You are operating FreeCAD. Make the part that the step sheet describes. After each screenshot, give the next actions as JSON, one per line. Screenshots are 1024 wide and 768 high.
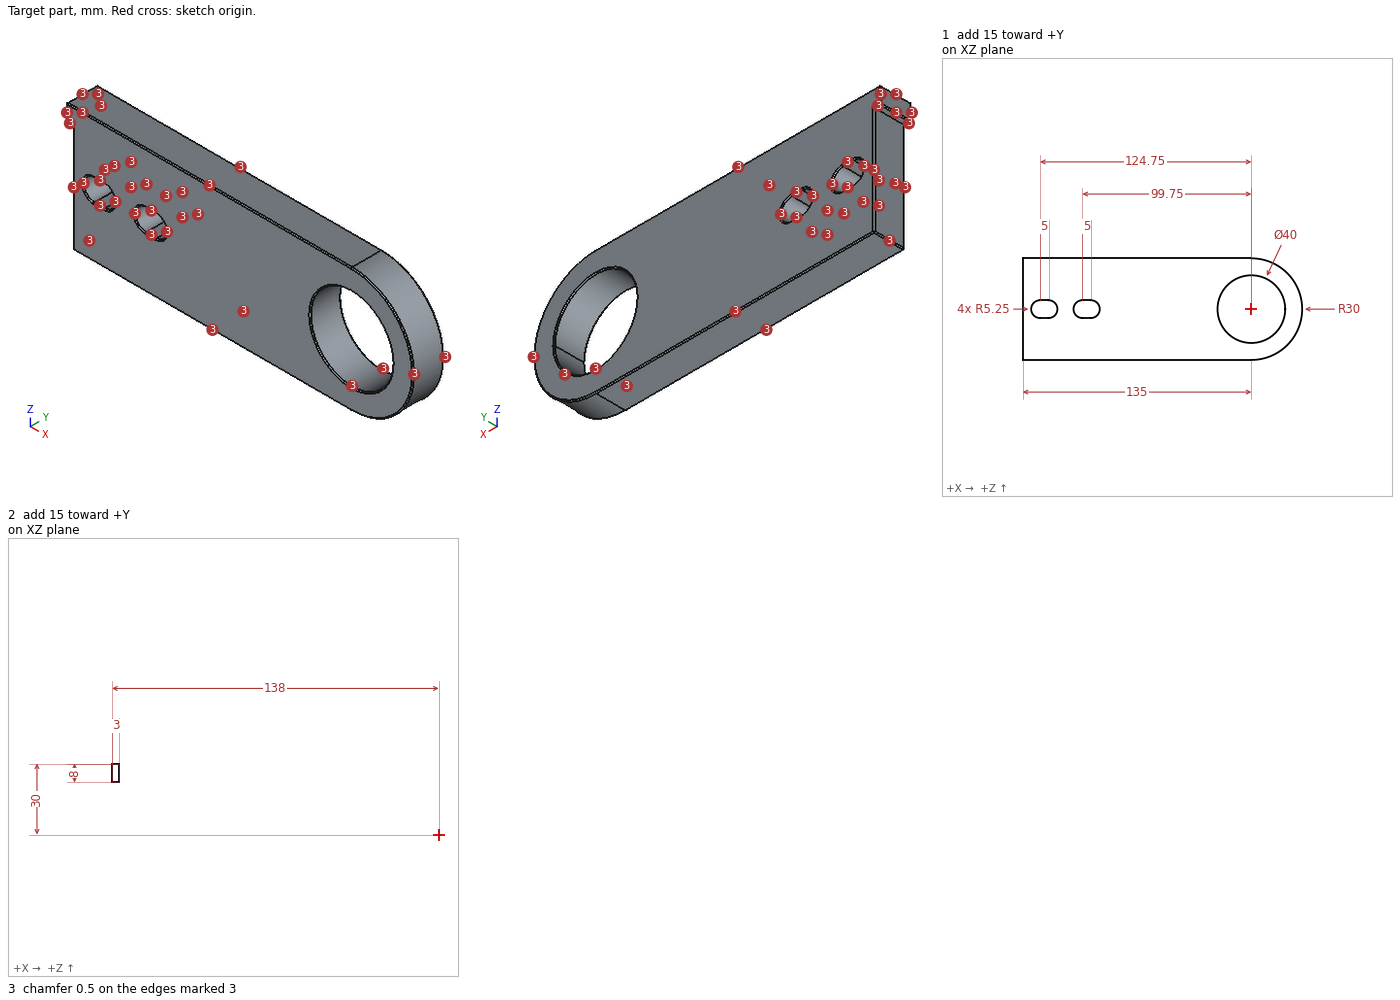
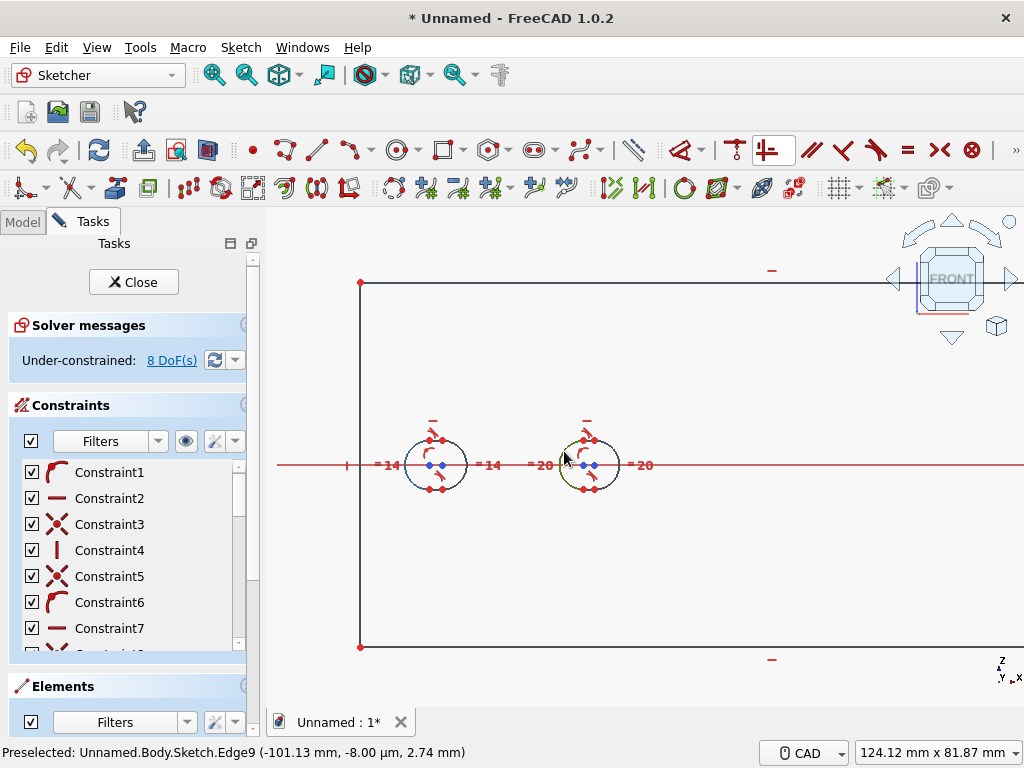
{"action": "left_click", "coordinate": [908, 150]}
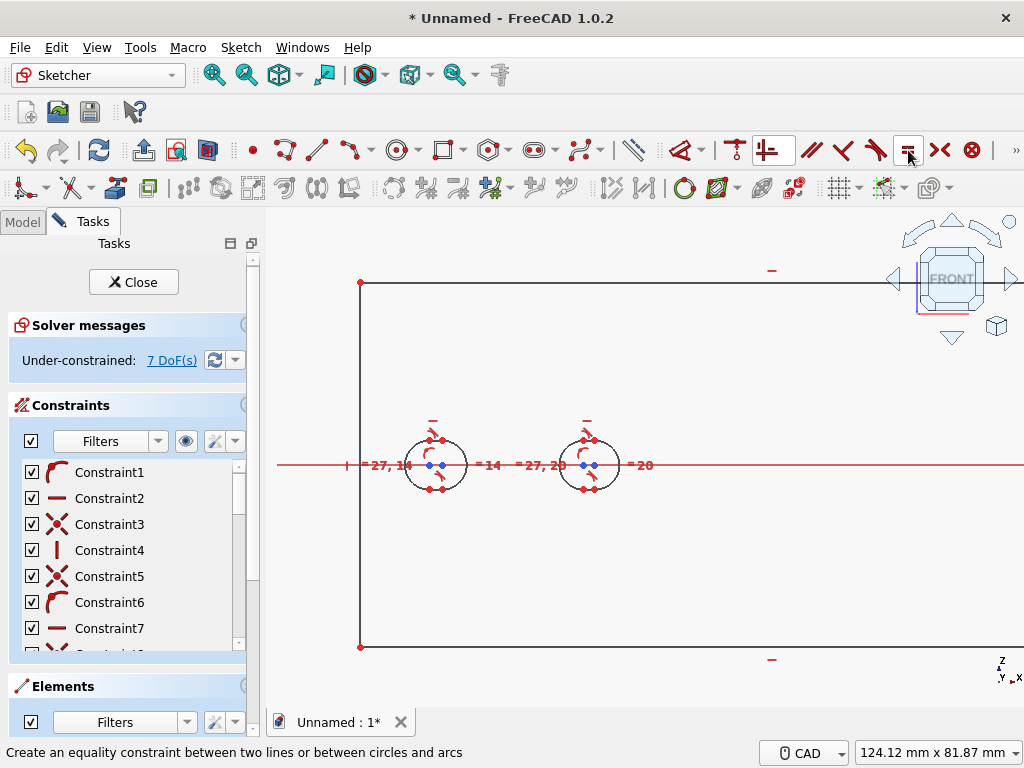
{"action": "left_click", "coordinate": [680, 150]}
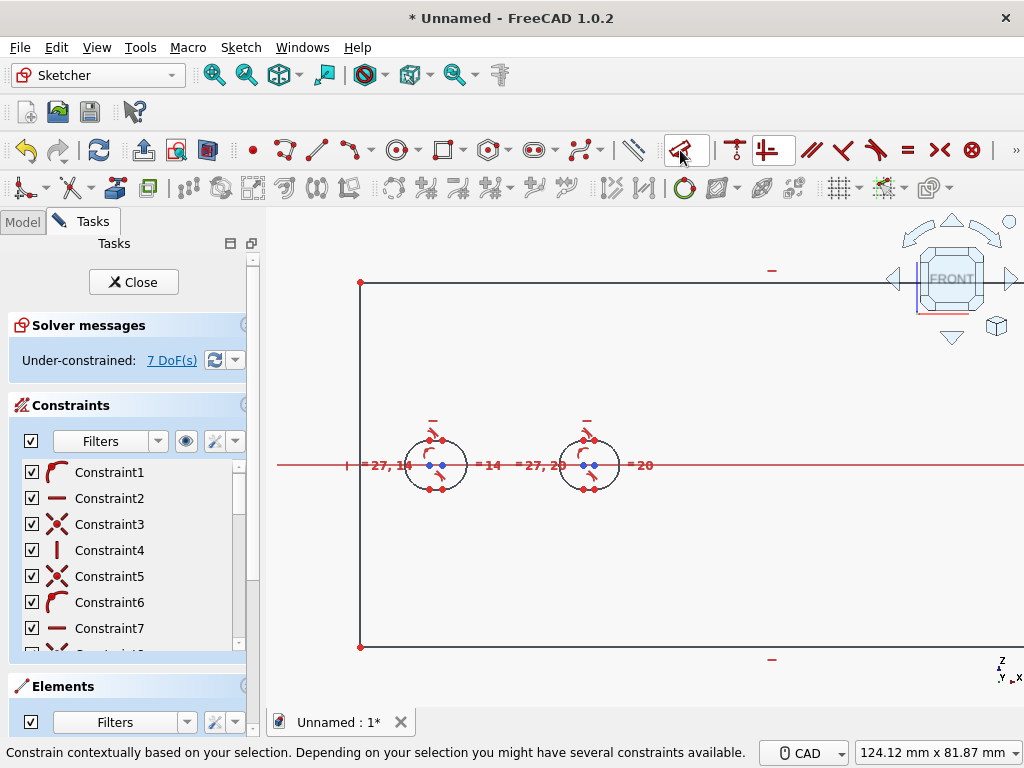
{"action": "scroll", "coordinate": [410, 452], "scroll_direction": "down", "scroll_amount": 5}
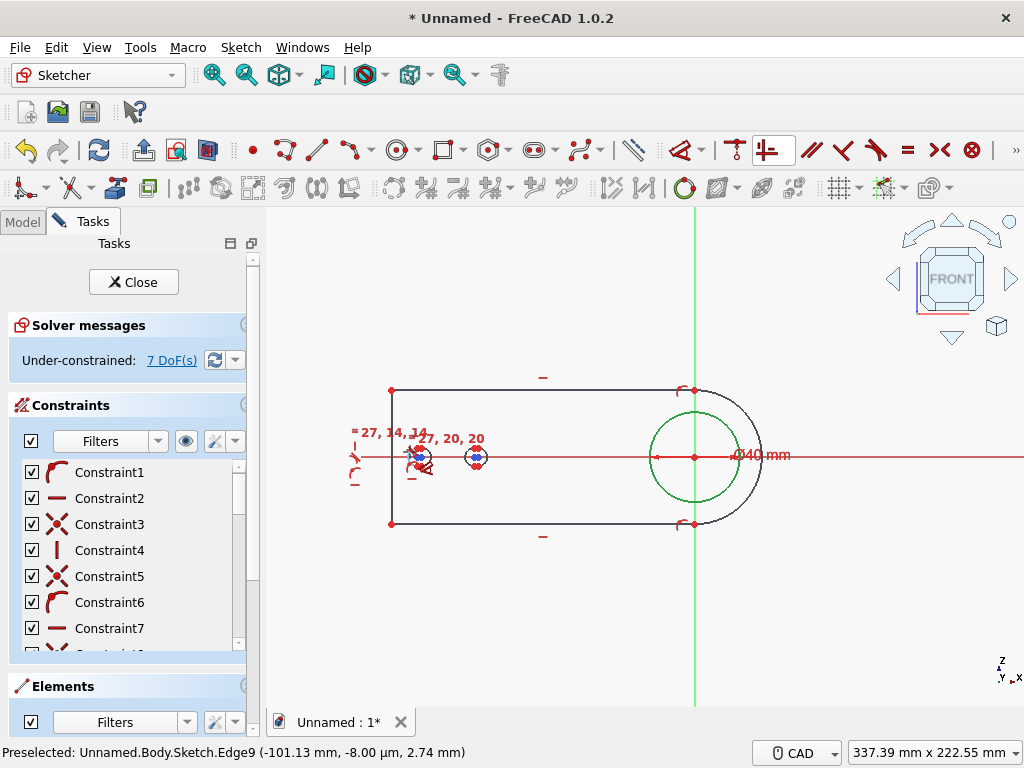
{"action": "left_click", "coordinate": [749, 497]}
{"action": "left_click", "coordinate": [775, 516]}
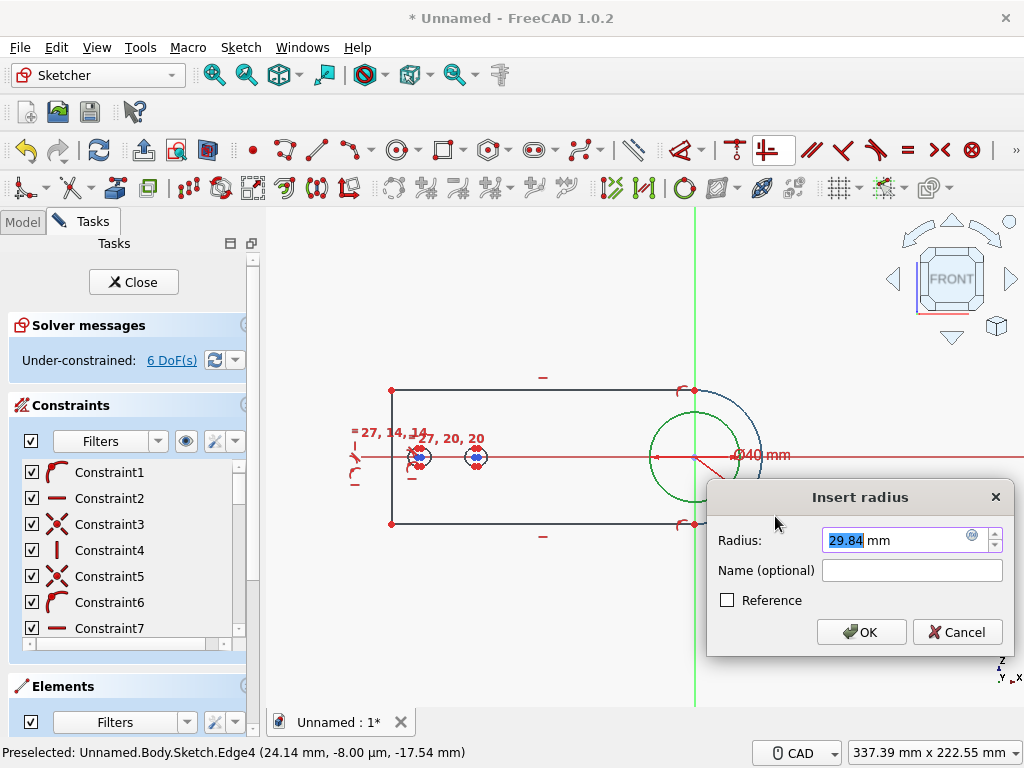
{"action": "type", "text": "30"}
{"action": "key", "text": "Return"}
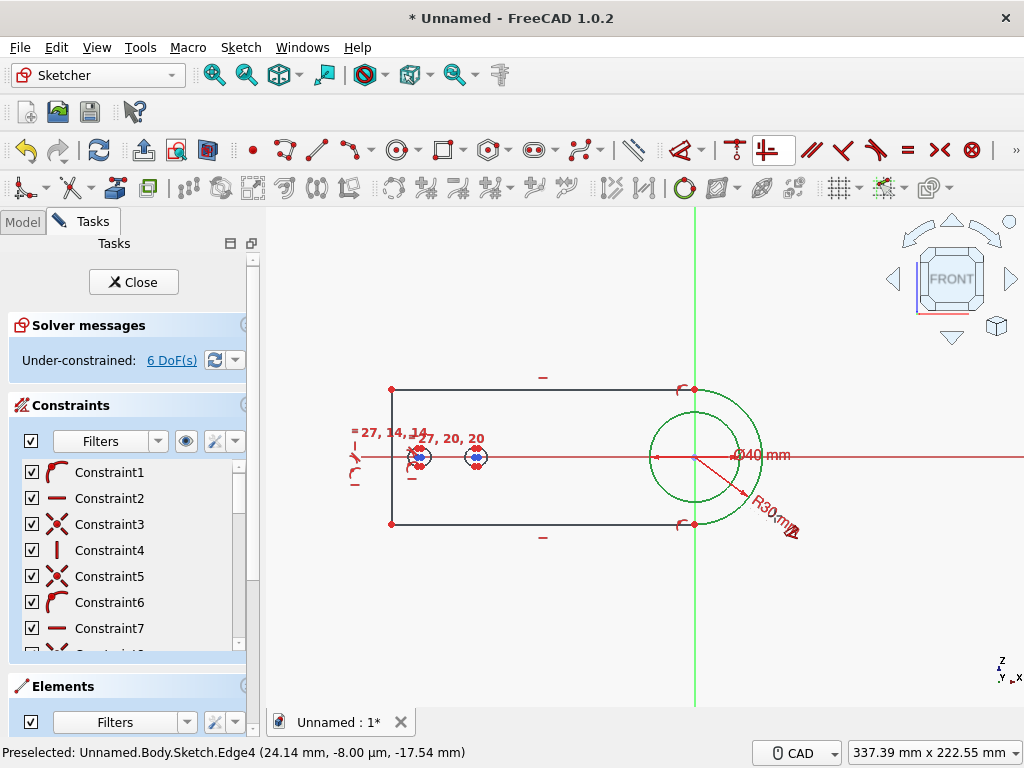
{"action": "scroll", "coordinate": [408, 457], "scroll_direction": "up", "scroll_amount": 7}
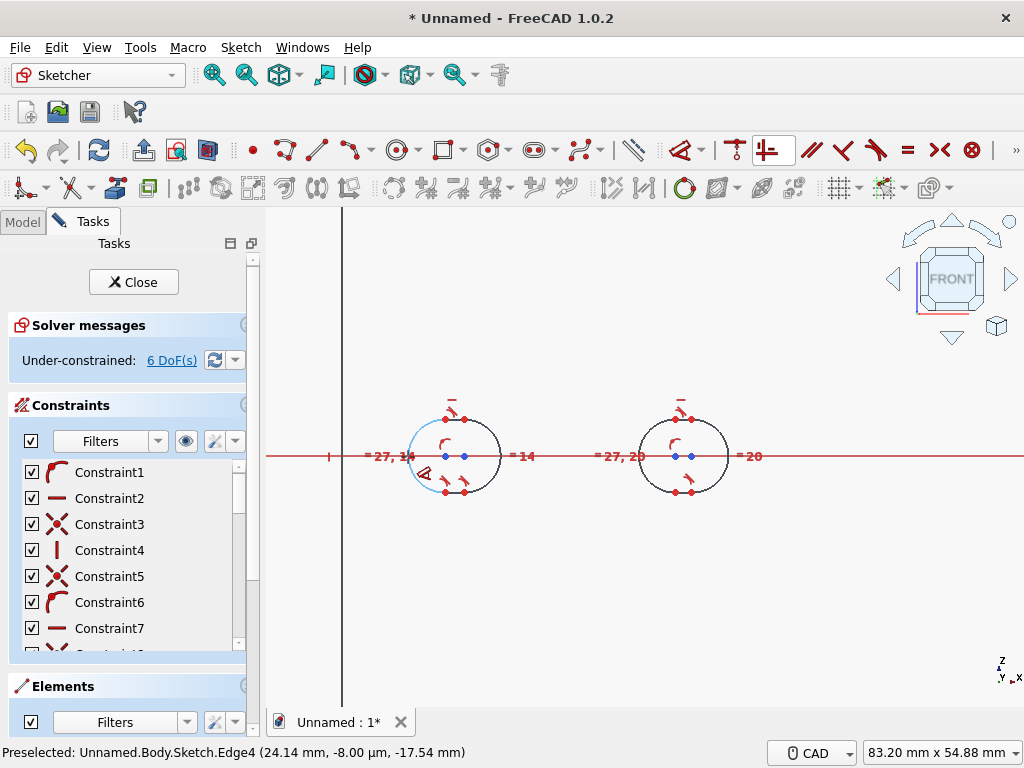
{"action": "left_click", "coordinate": [409, 456]}
{"action": "left_click", "coordinate": [385, 423]}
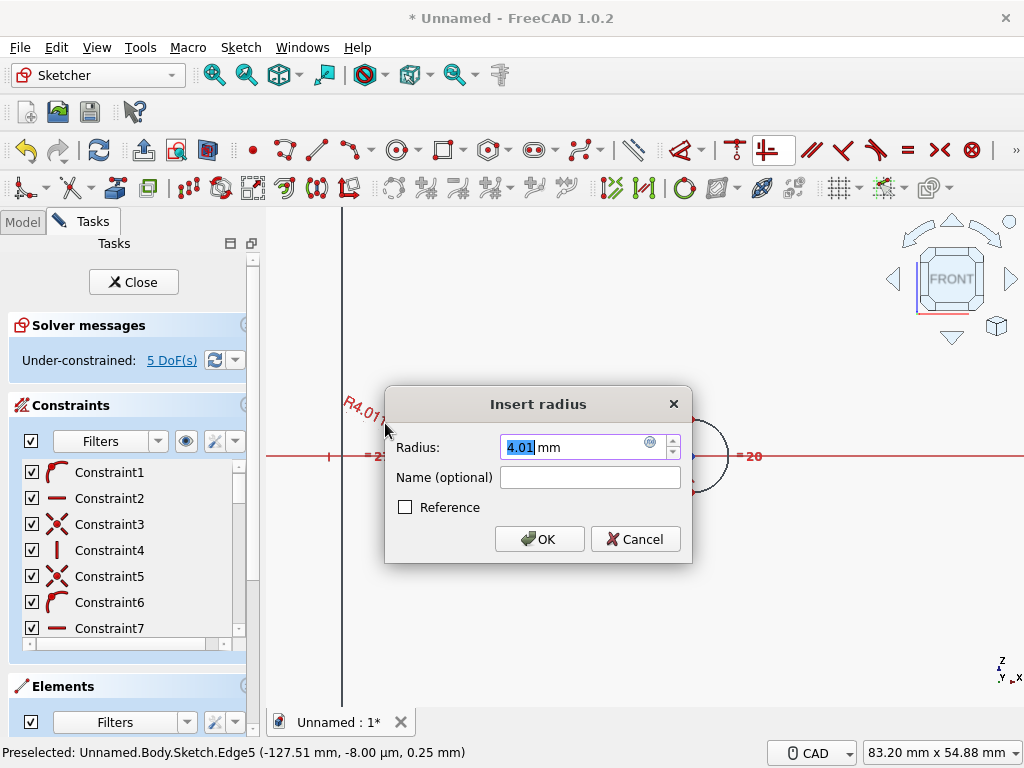
{"action": "type", "text": "5.25"}
{"action": "key", "text": "Return"}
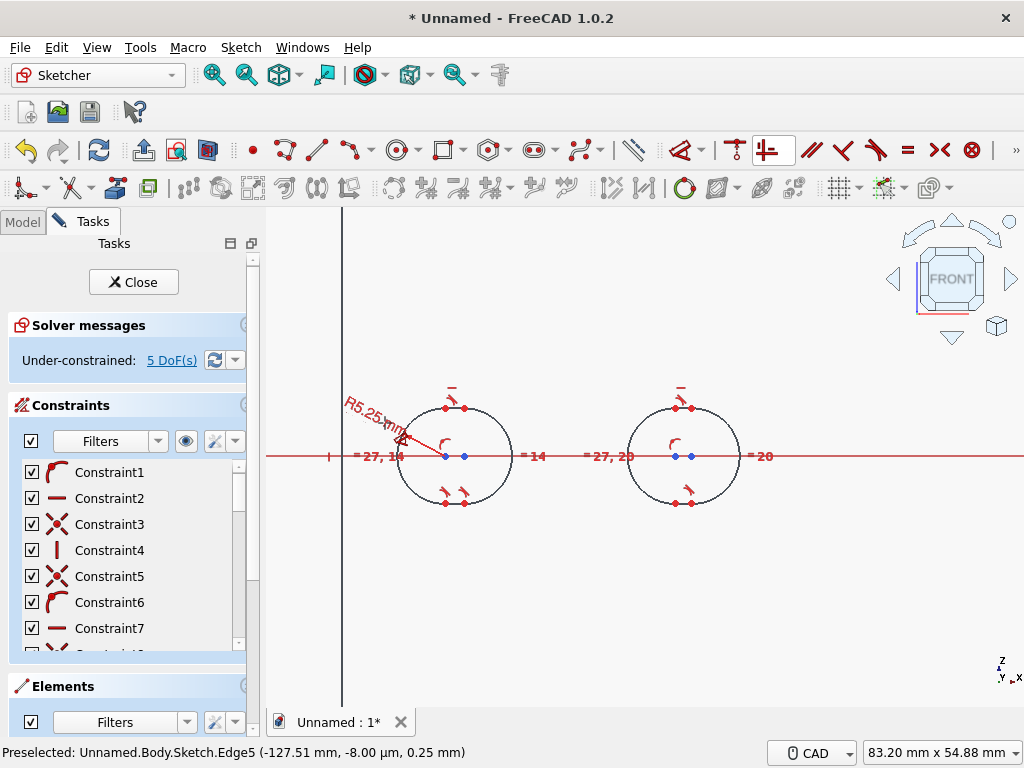
{"action": "scroll", "coordinate": [455, 408], "scroll_direction": "up", "scroll_amount": 2}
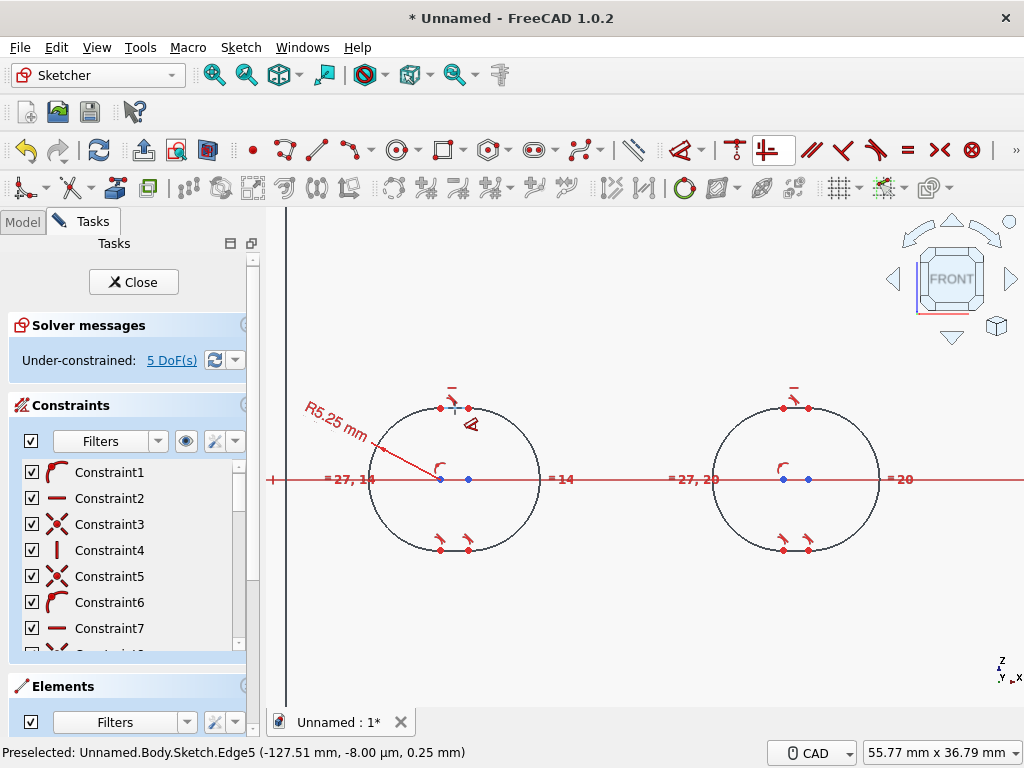
{"action": "left_click", "coordinate": [454, 408]}
{"action": "left_click", "coordinate": [454, 374]}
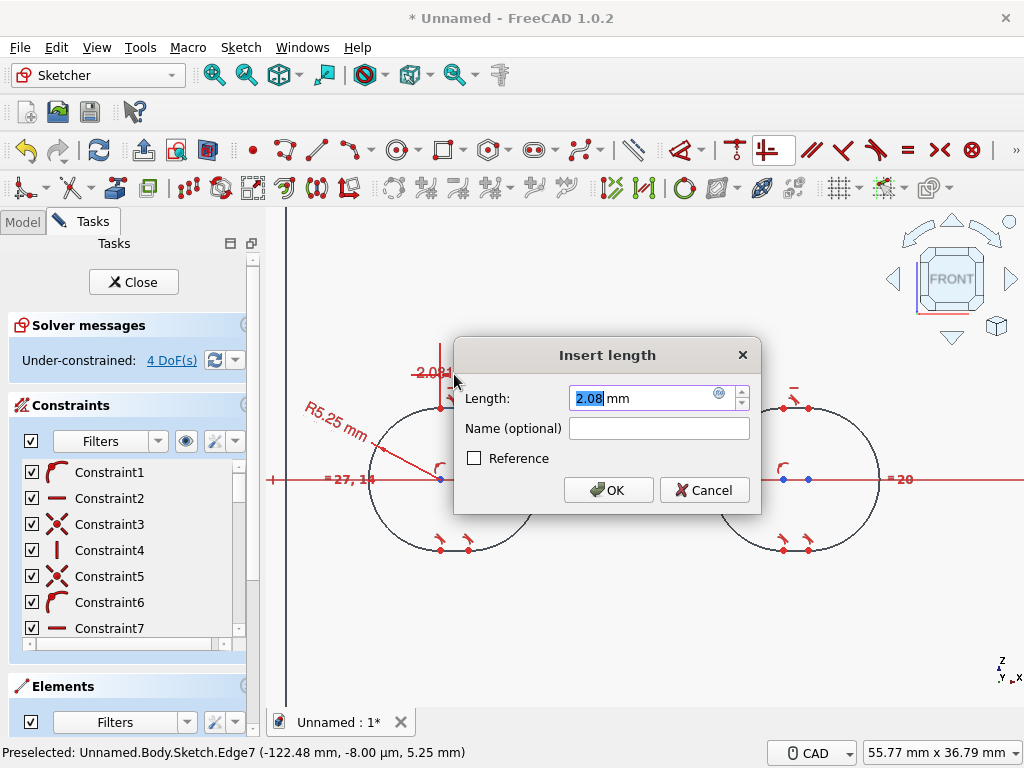
{"action": "type", "text": "5"}
{"action": "key", "text": "Return"}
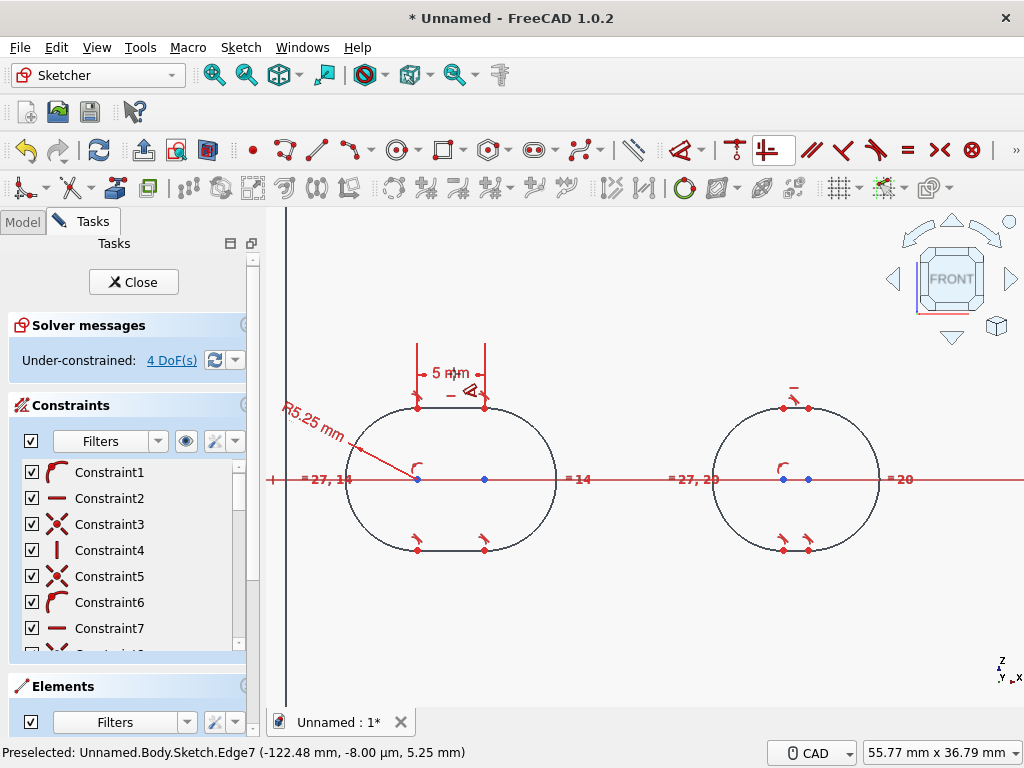
{"action": "scroll", "coordinate": [794, 408], "scroll_direction": "up", "scroll_amount": 2}